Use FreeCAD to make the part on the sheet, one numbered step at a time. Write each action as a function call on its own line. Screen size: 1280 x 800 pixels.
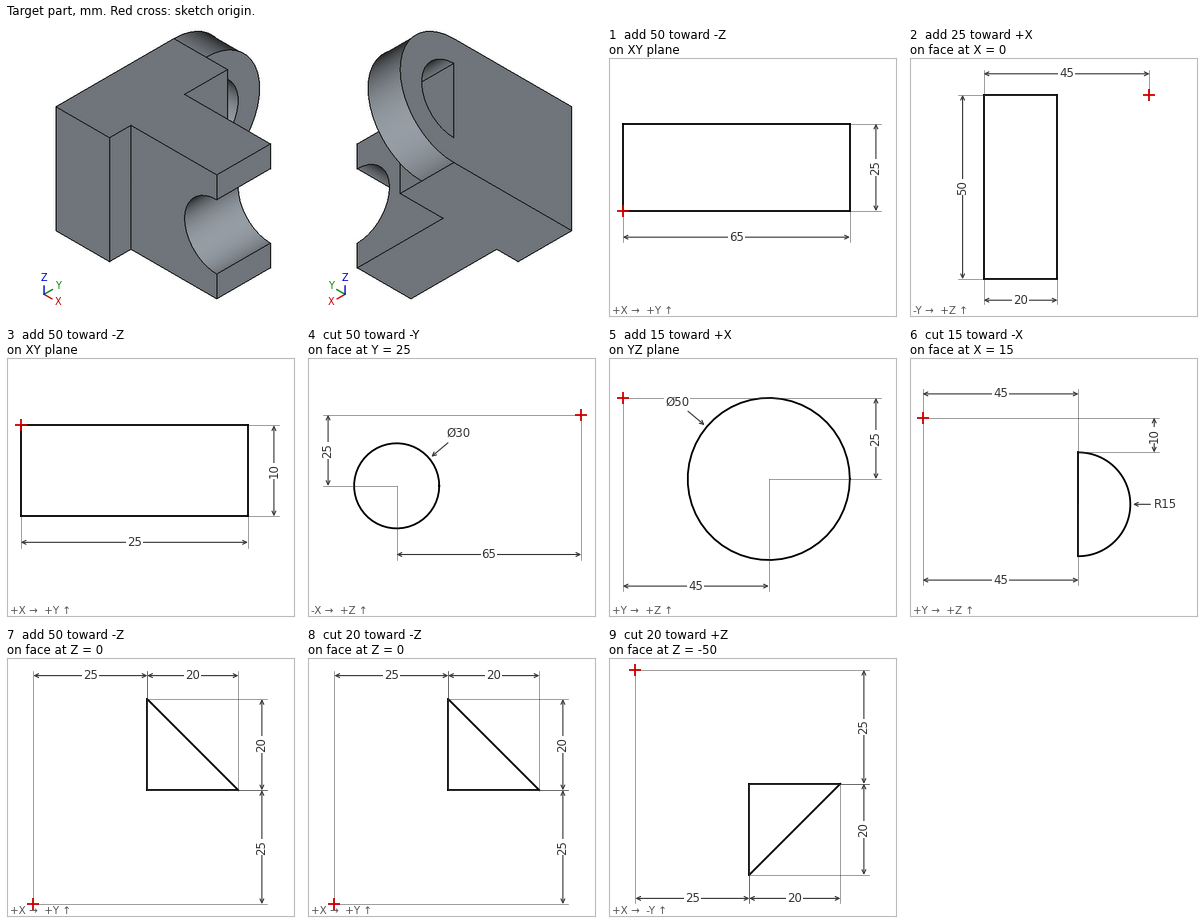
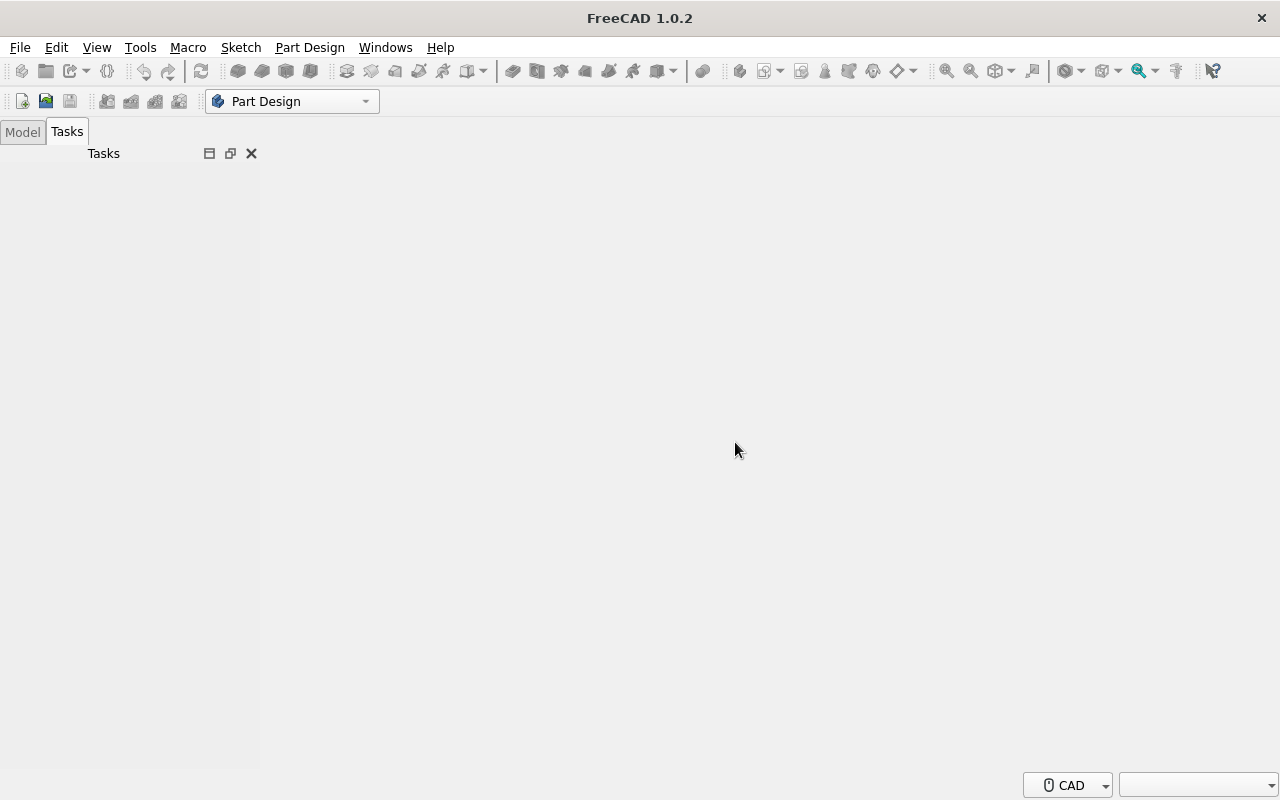
click(22, 102)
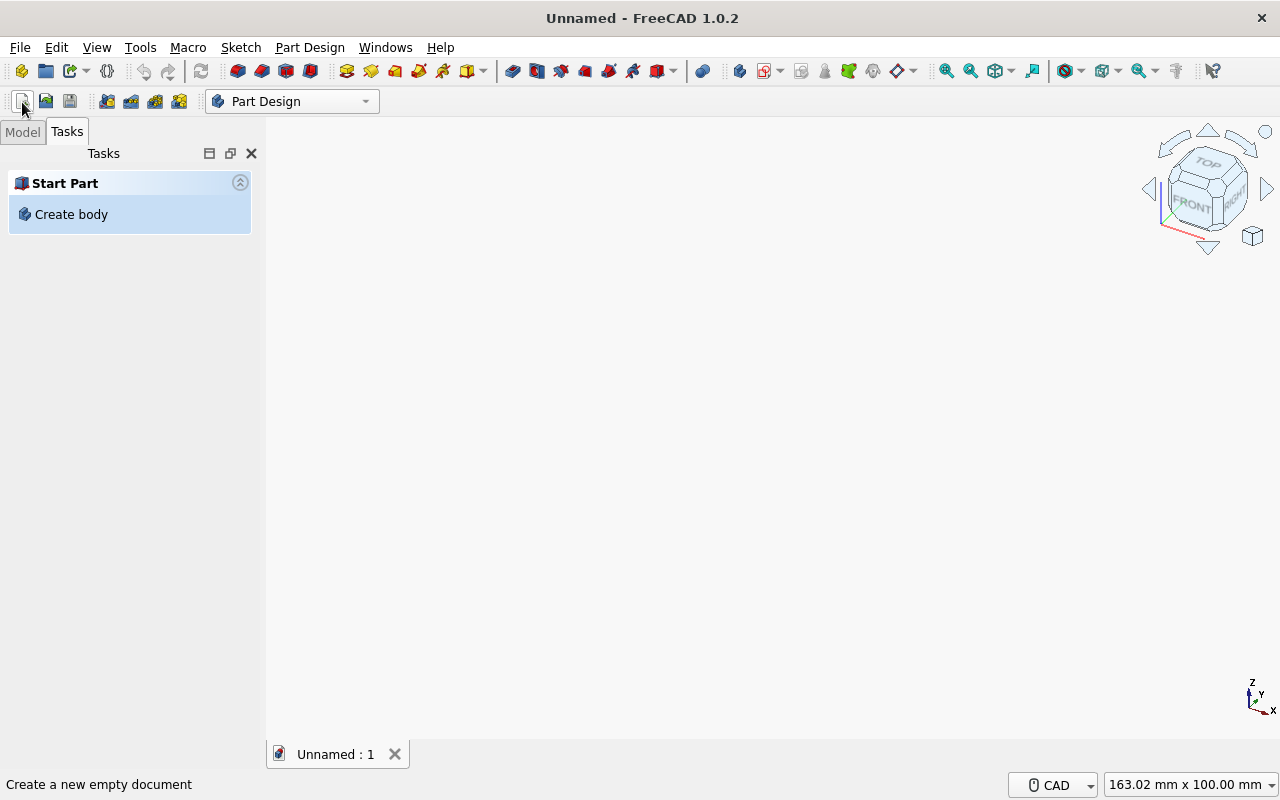
click(764, 72)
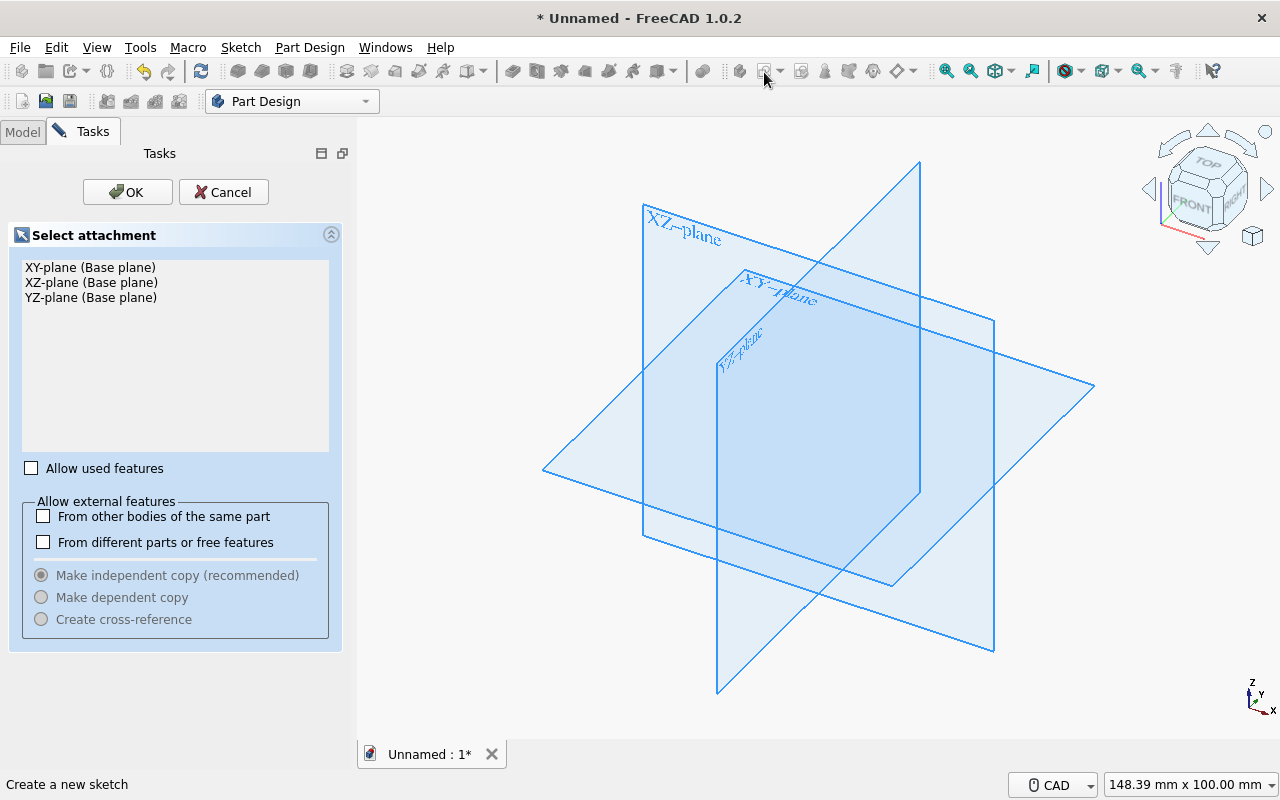
click(82, 268)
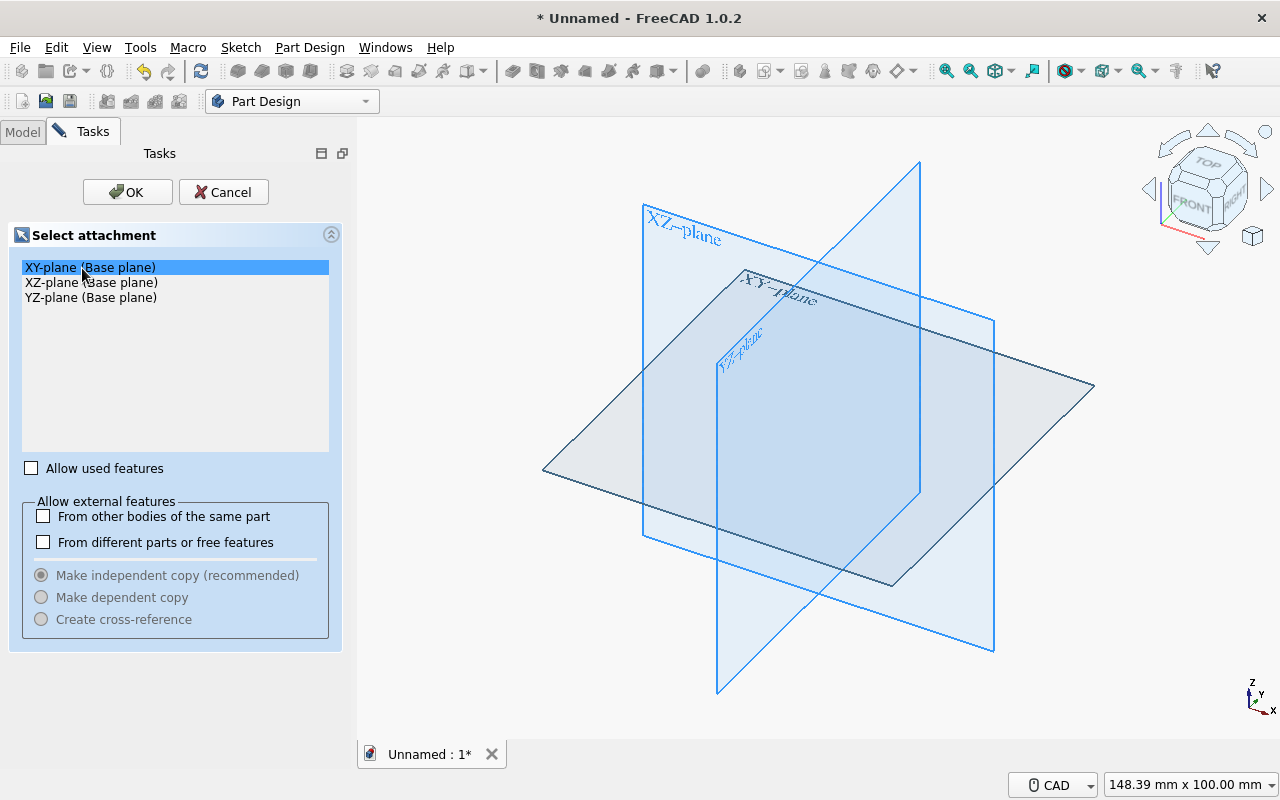
click(128, 192)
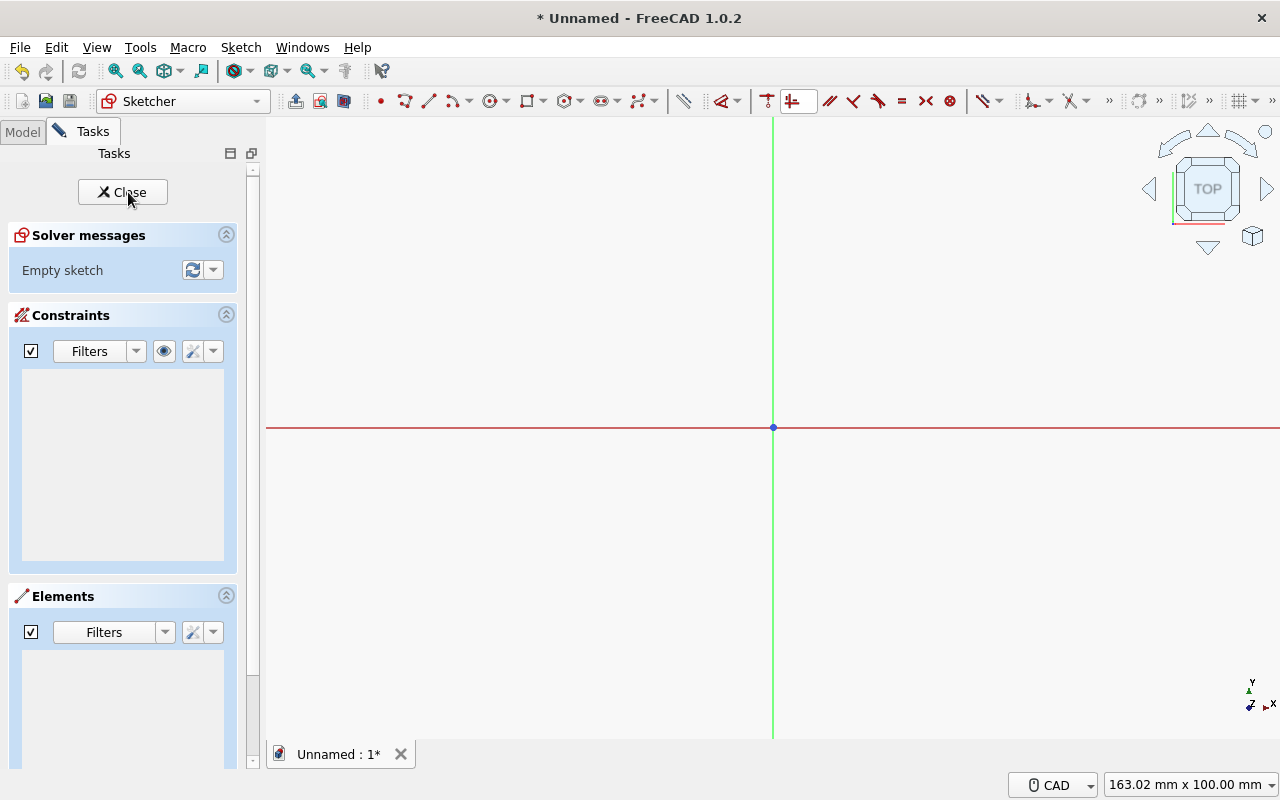
scroll(294, 711, down, 1)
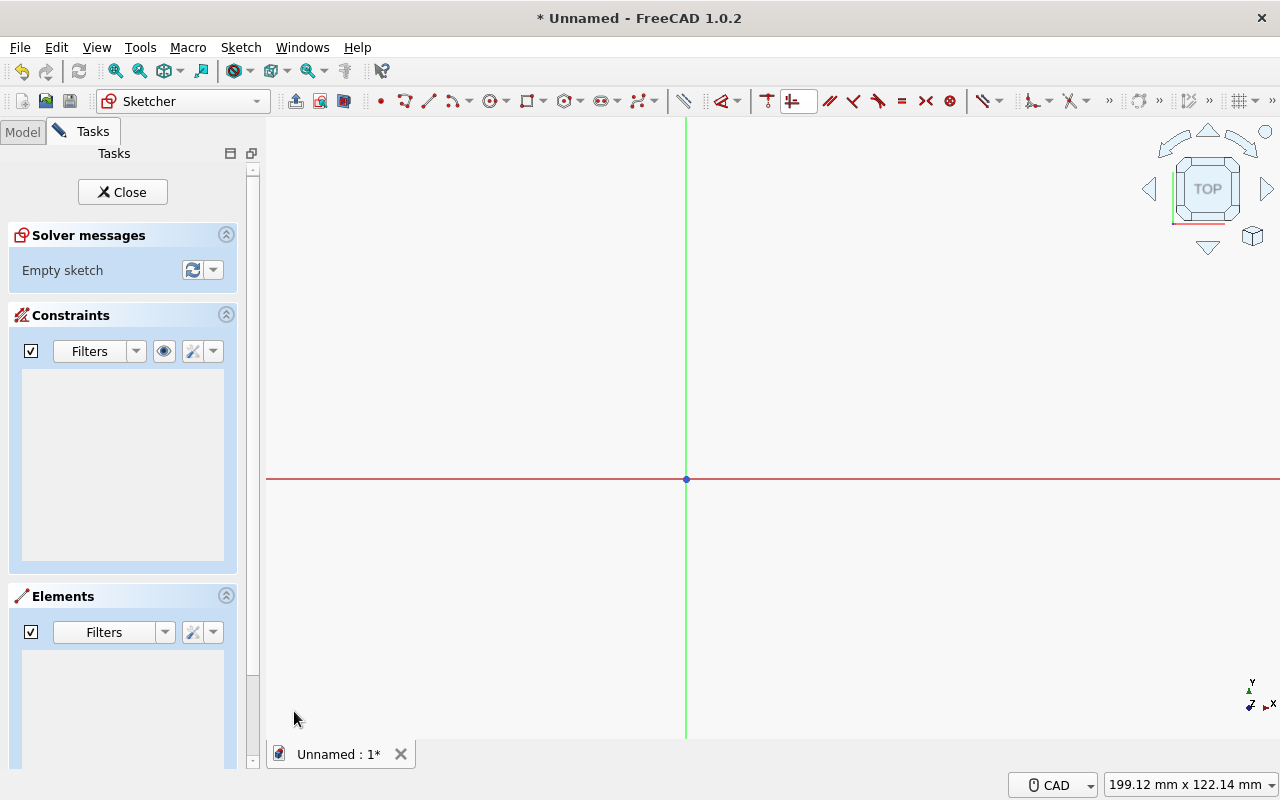
scroll(1031, 401, up, 3)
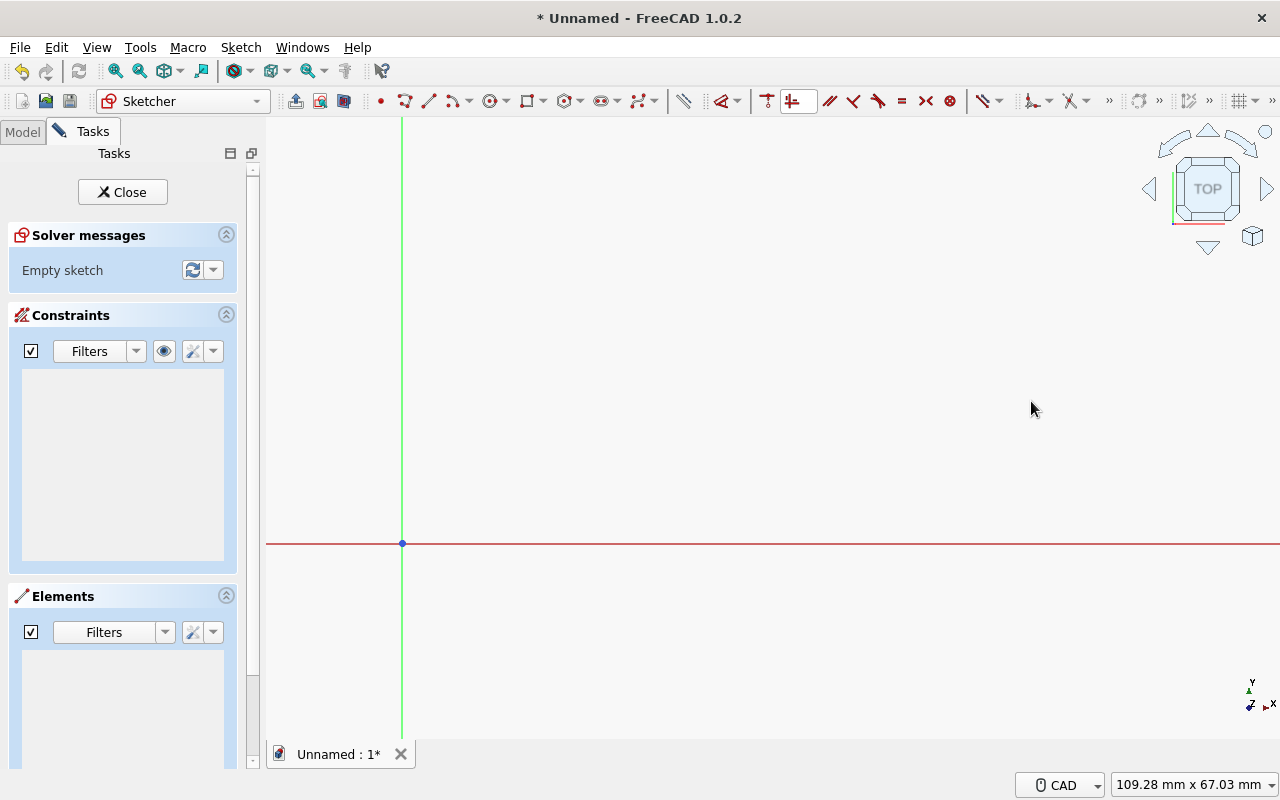
click(528, 102)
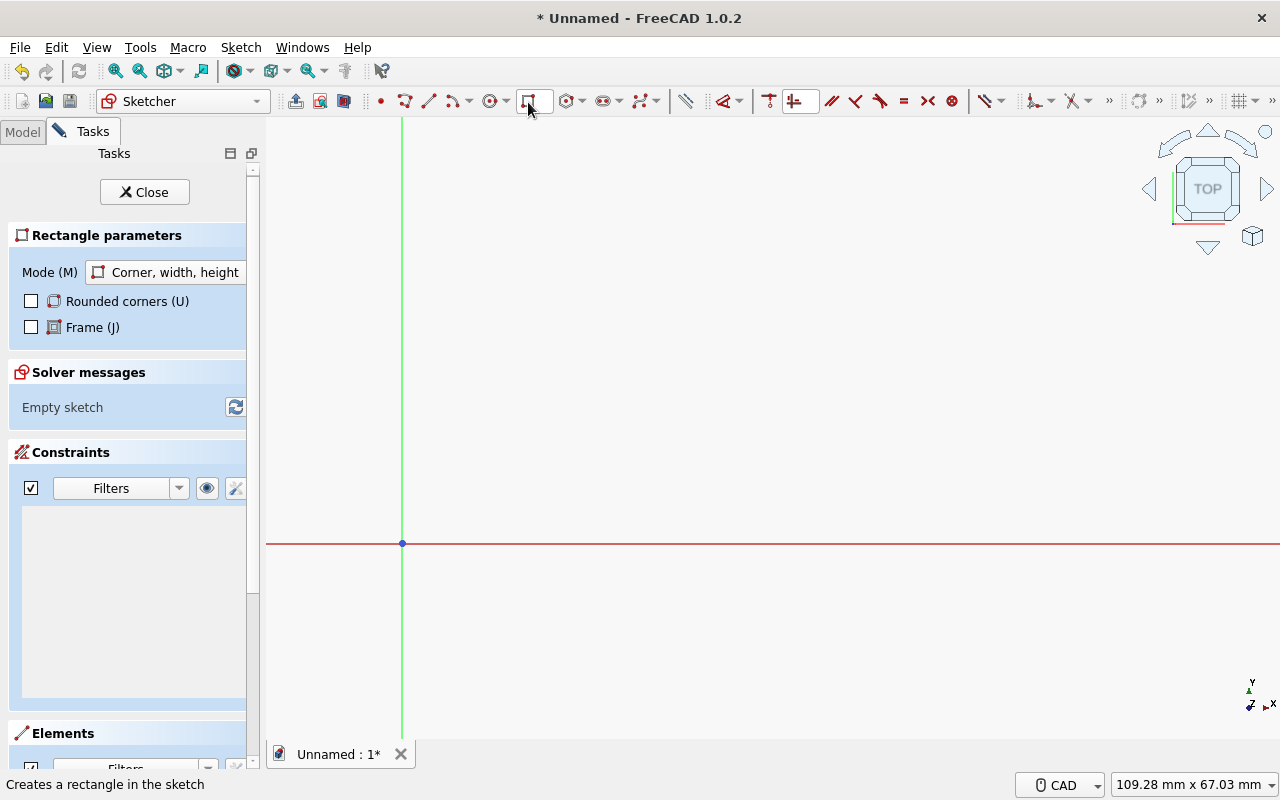
click(402, 544)
move(1005, 312)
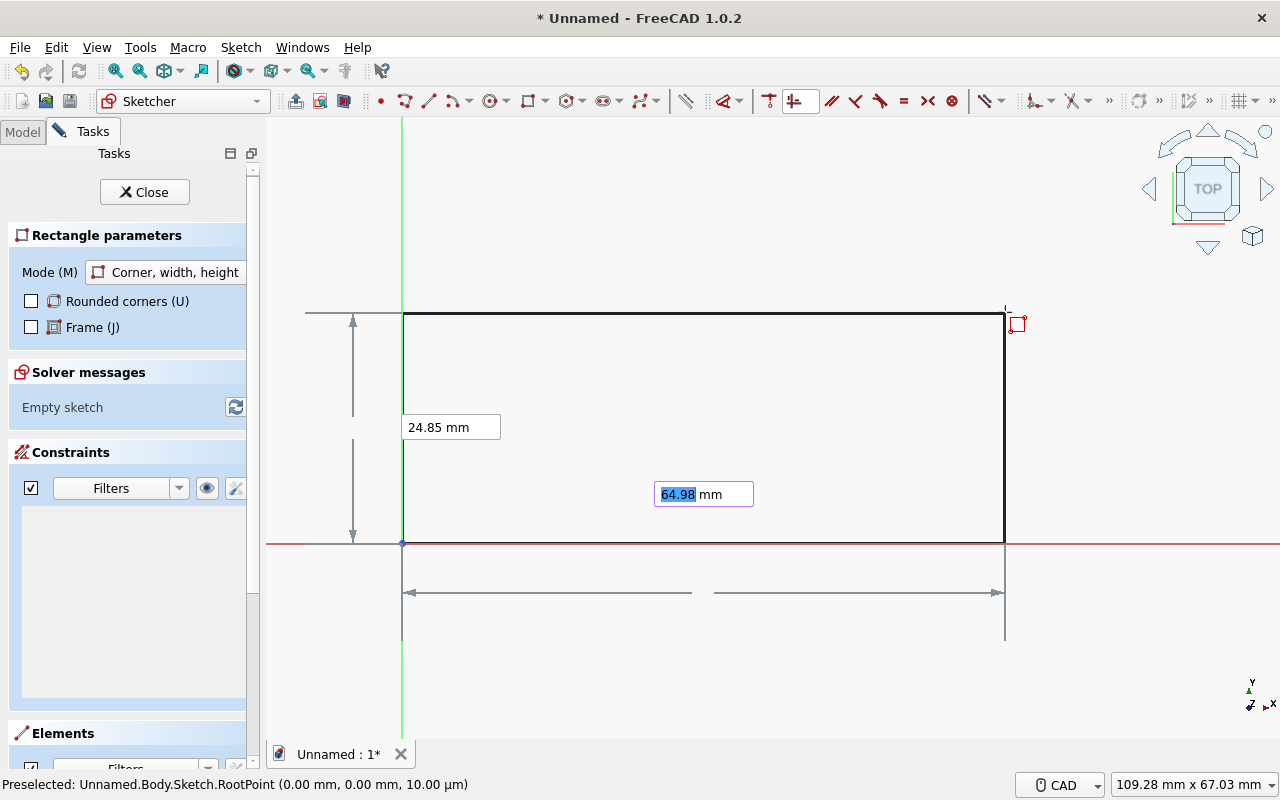
text(65)
key(Tab)
text(25)
key(Return)
key(Escape)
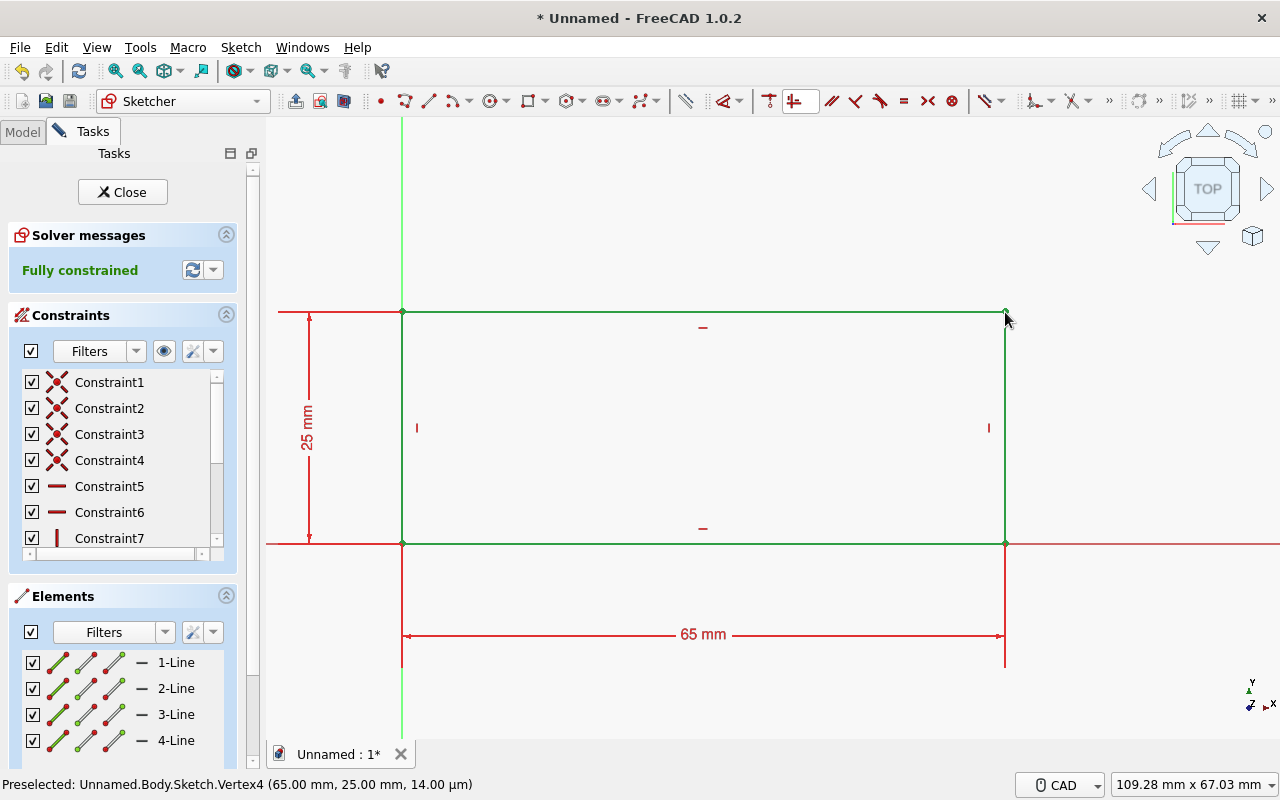
click(123, 192)